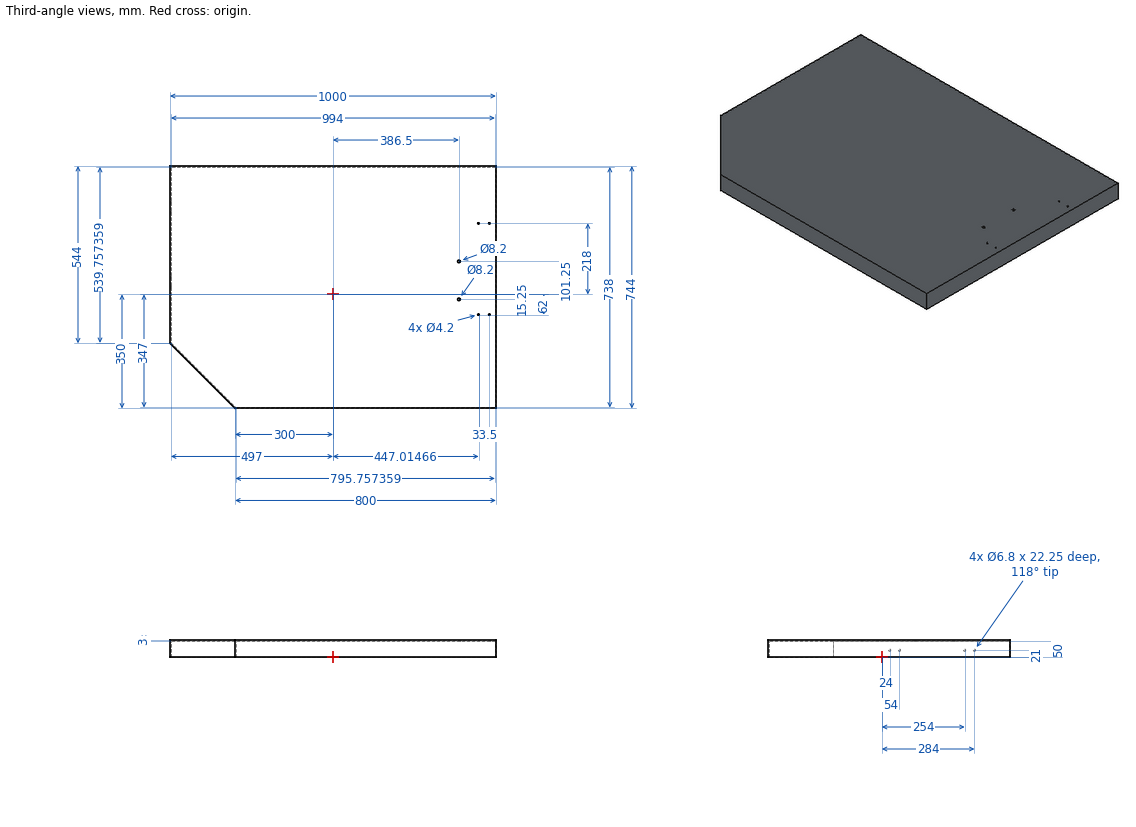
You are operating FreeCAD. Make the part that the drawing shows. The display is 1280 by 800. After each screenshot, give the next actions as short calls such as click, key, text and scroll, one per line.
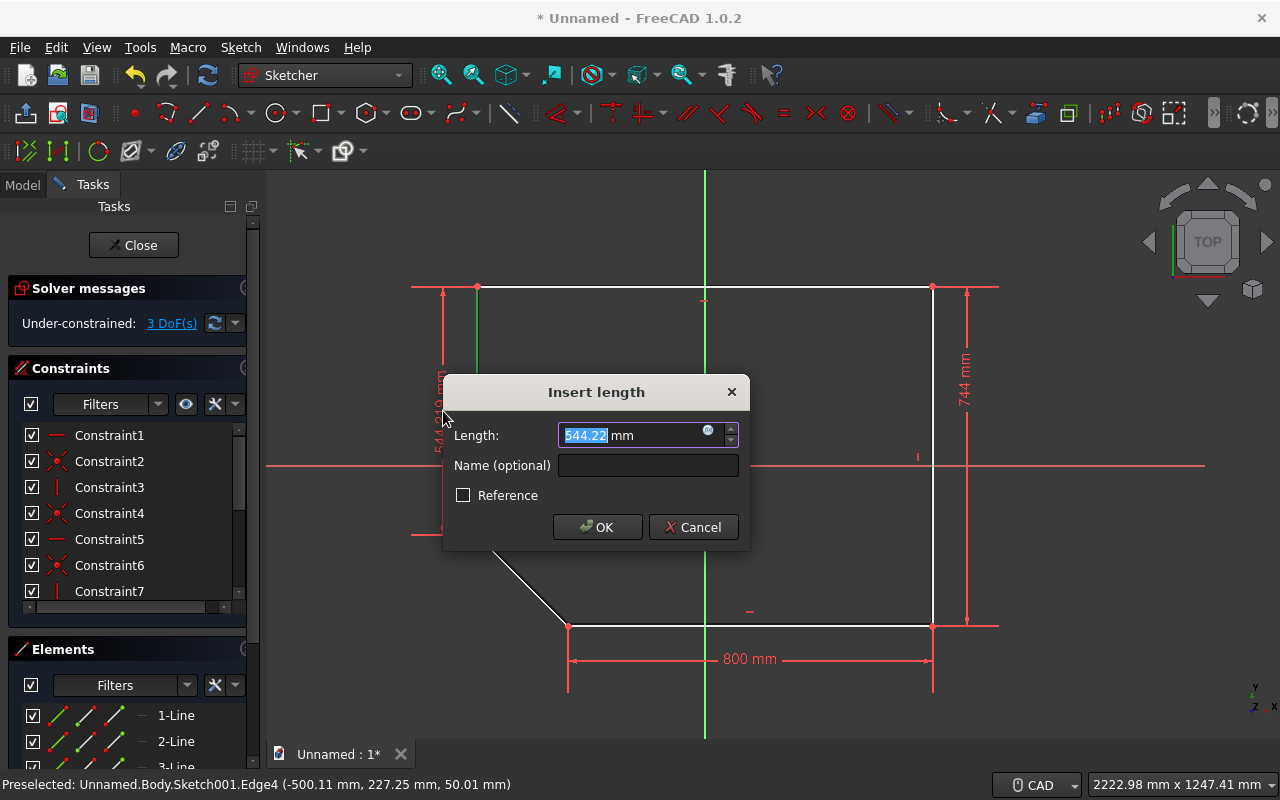
text(544)
key(Return)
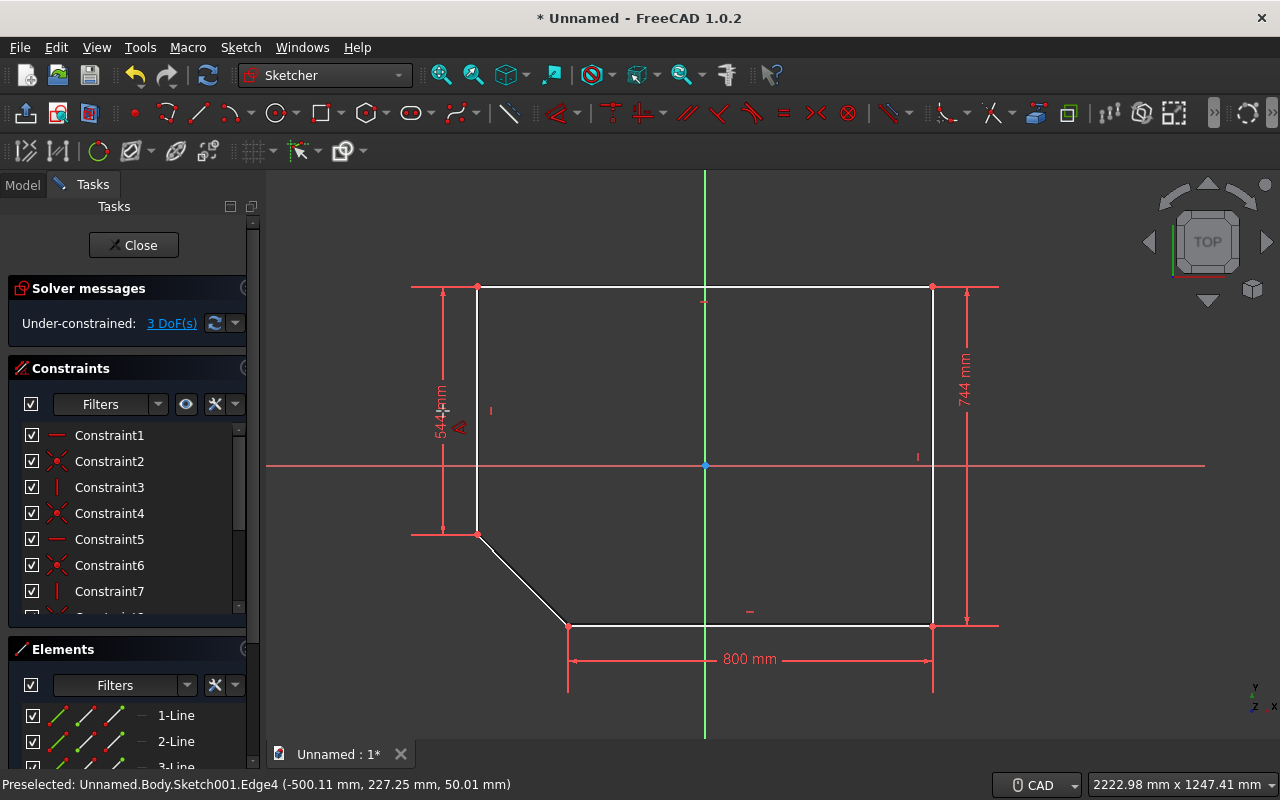
click(796, 287)
click(600, 253)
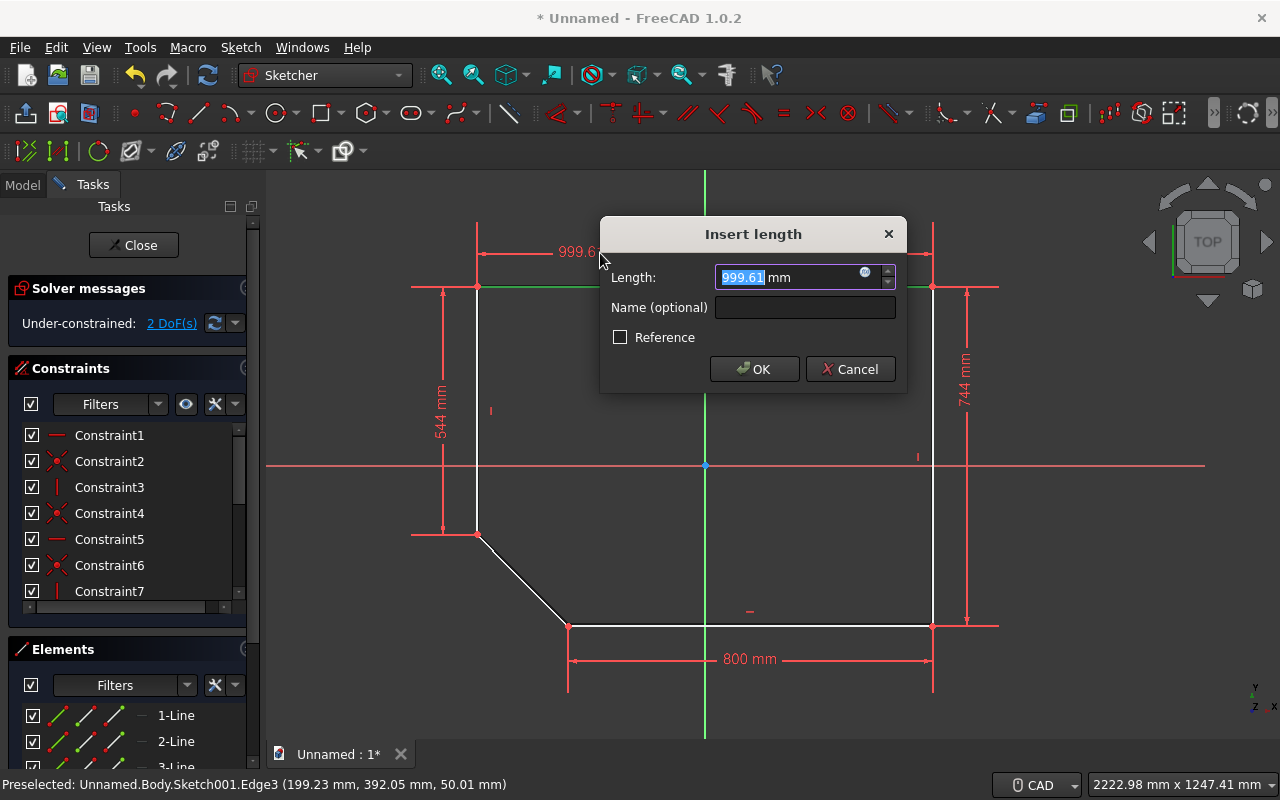
text(1000)
key(Return)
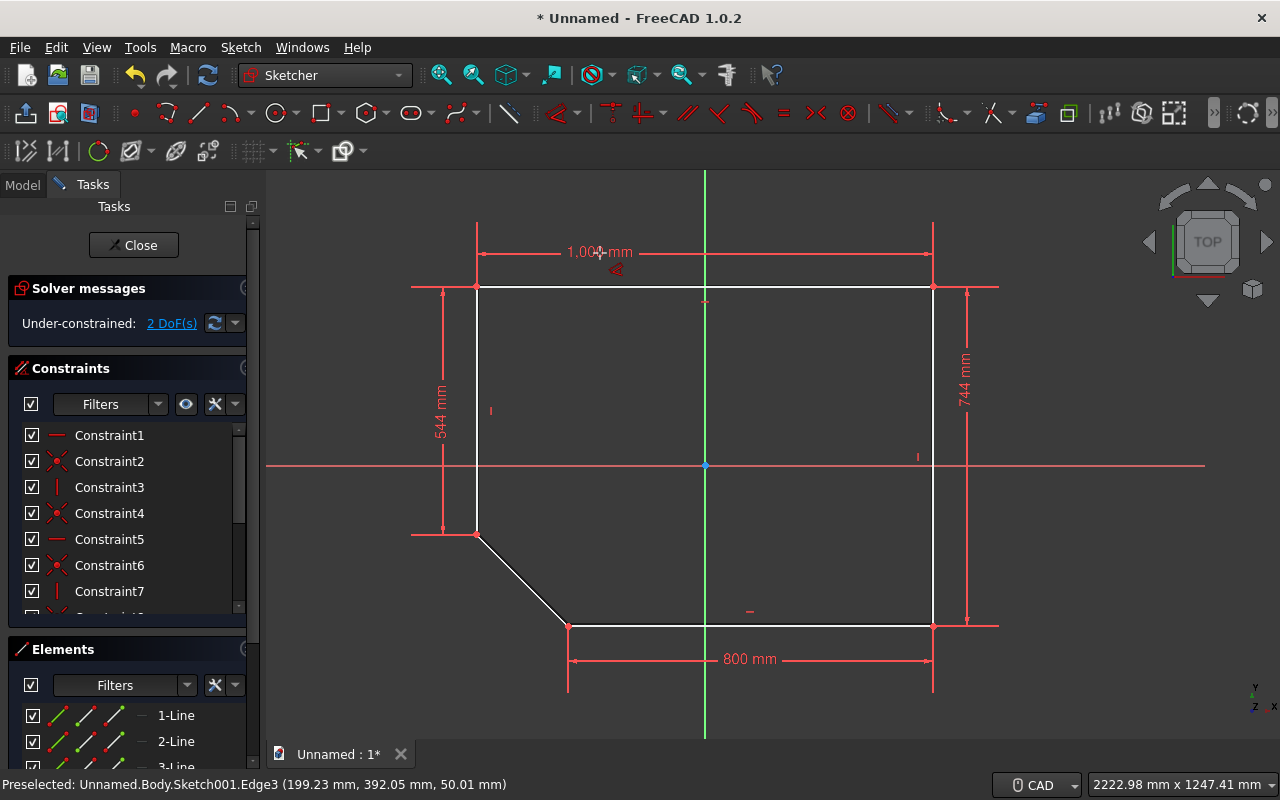
click(568, 626)
click(637, 660)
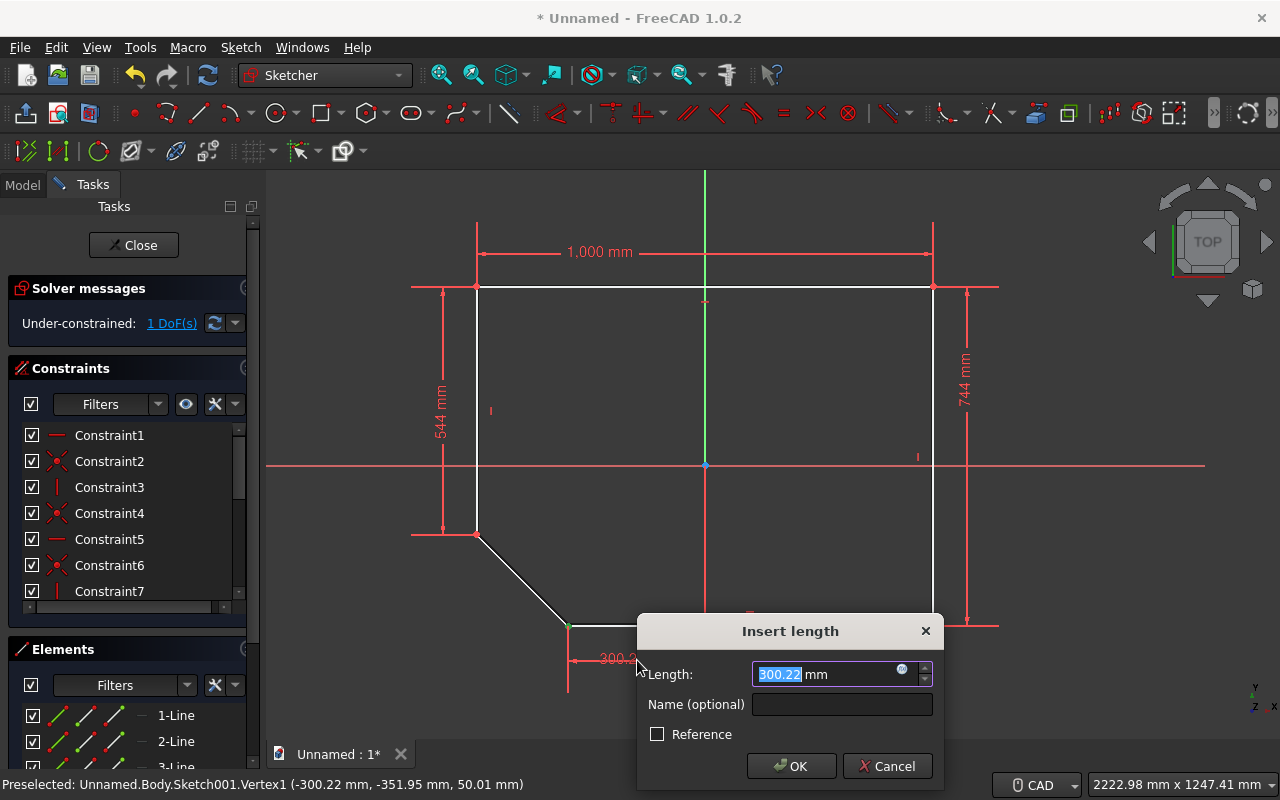
text(300)
key(Return)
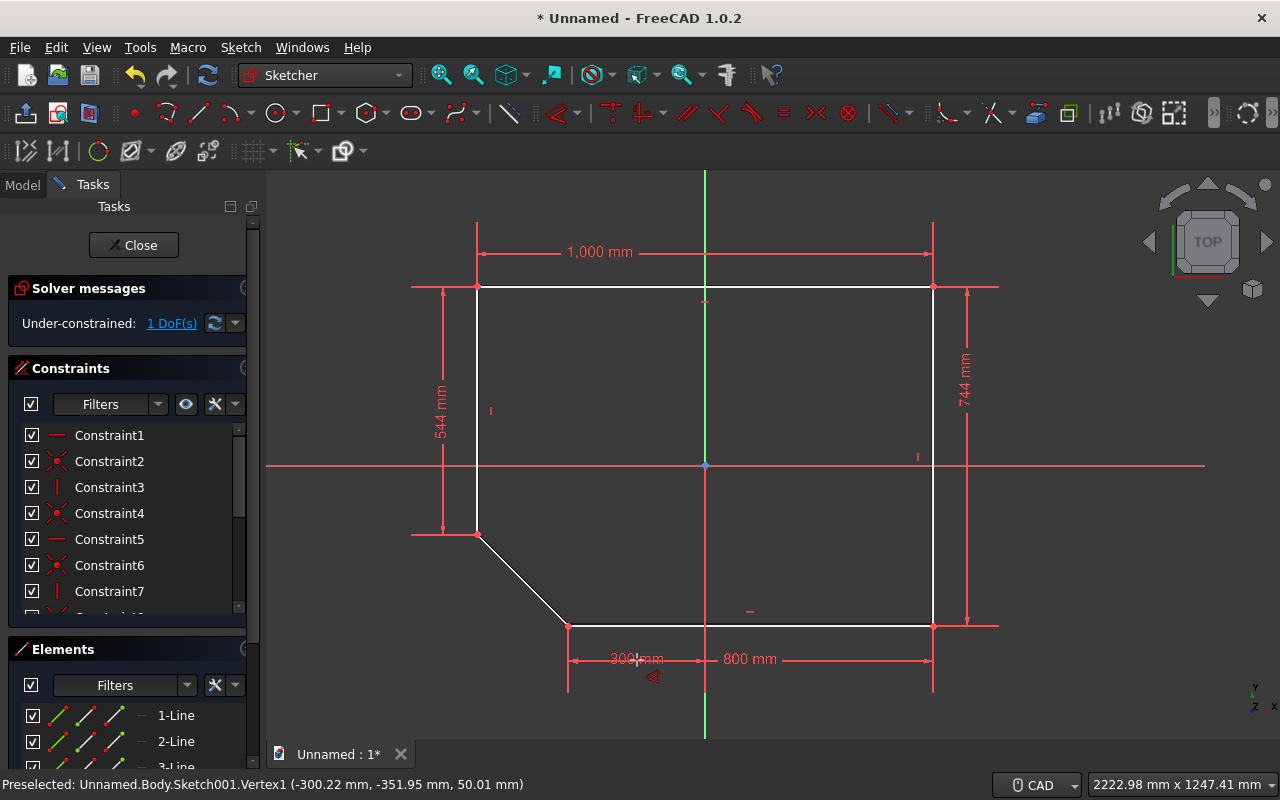
click(568, 626)
click(534, 546)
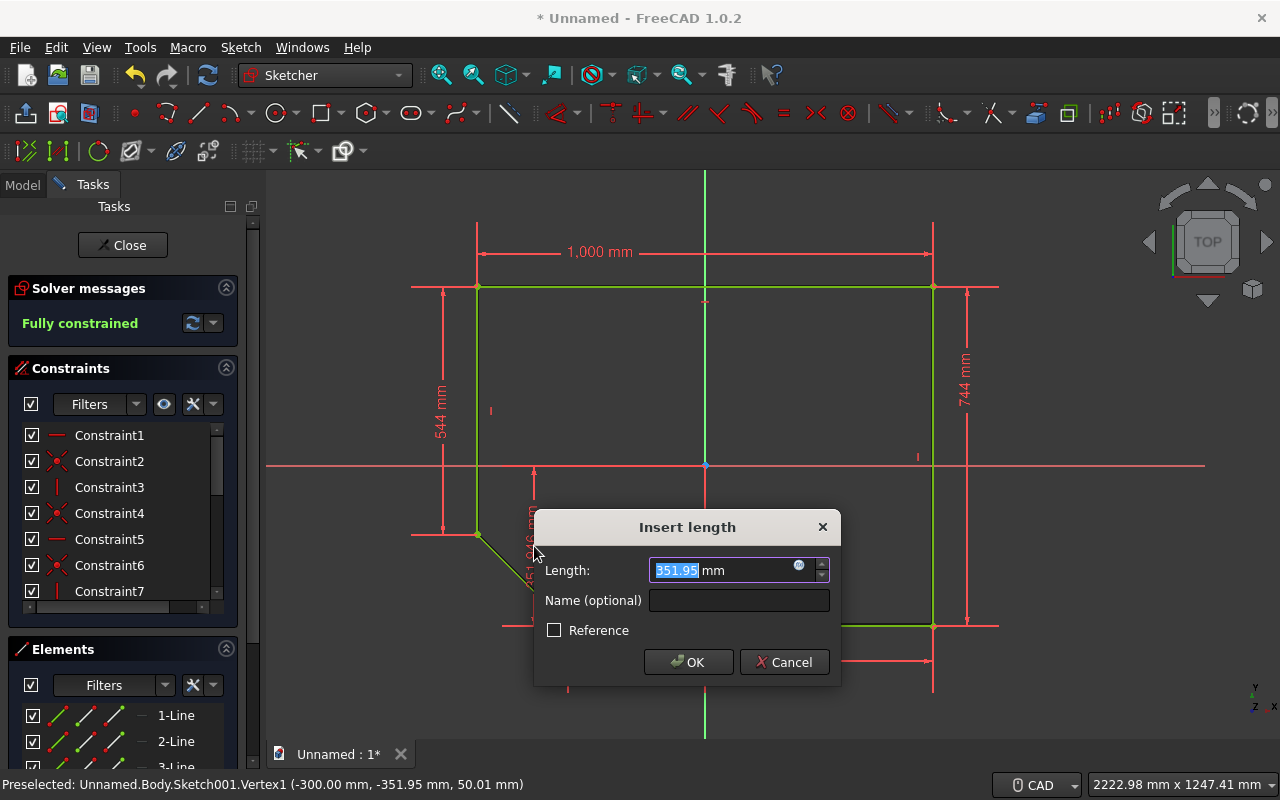
text(350)
key(Return)
key(Escape)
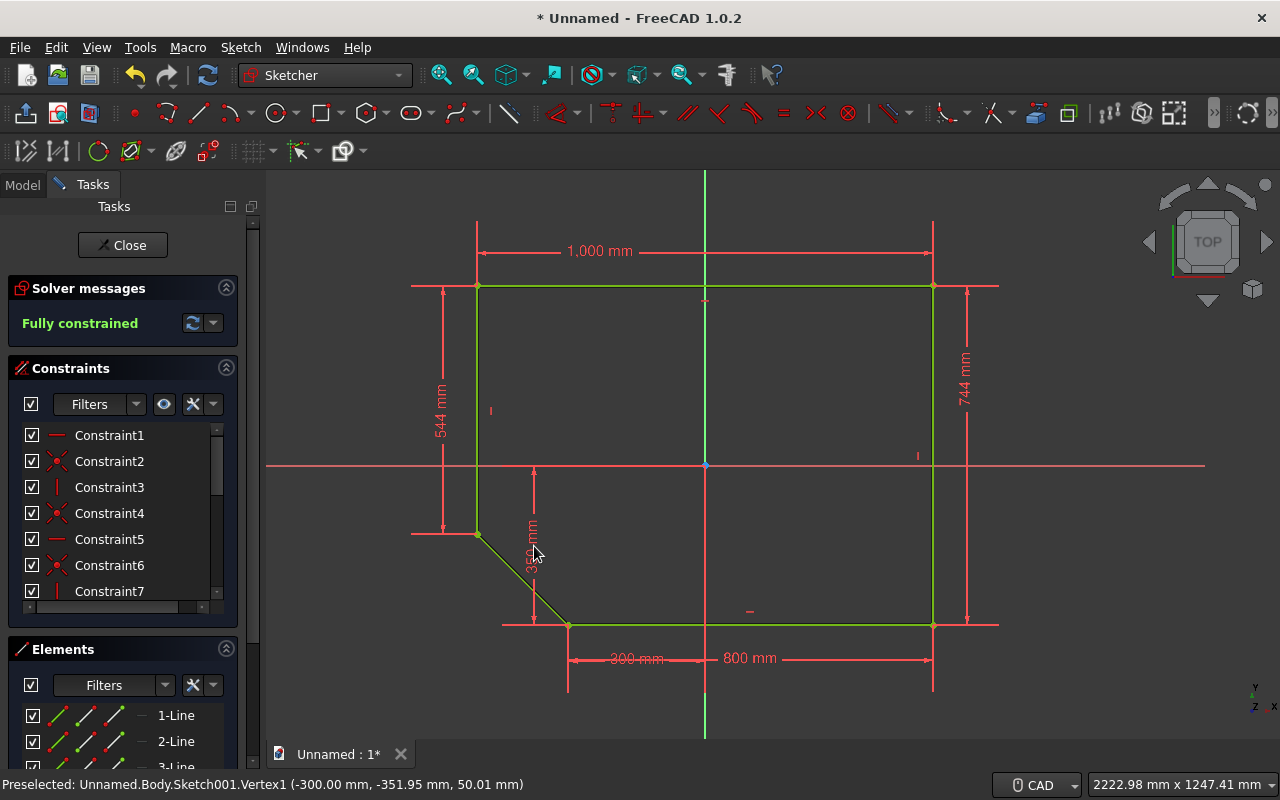
click(123, 245)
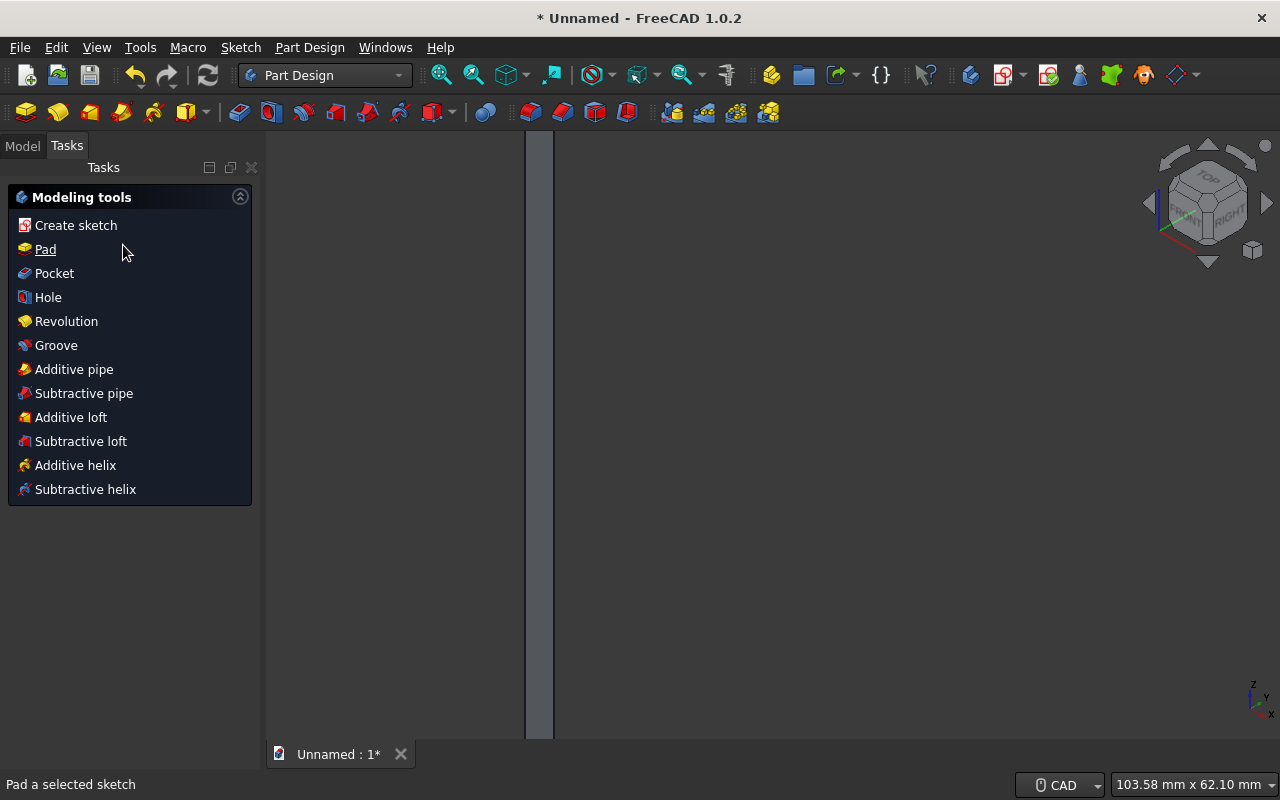
click(26, 112)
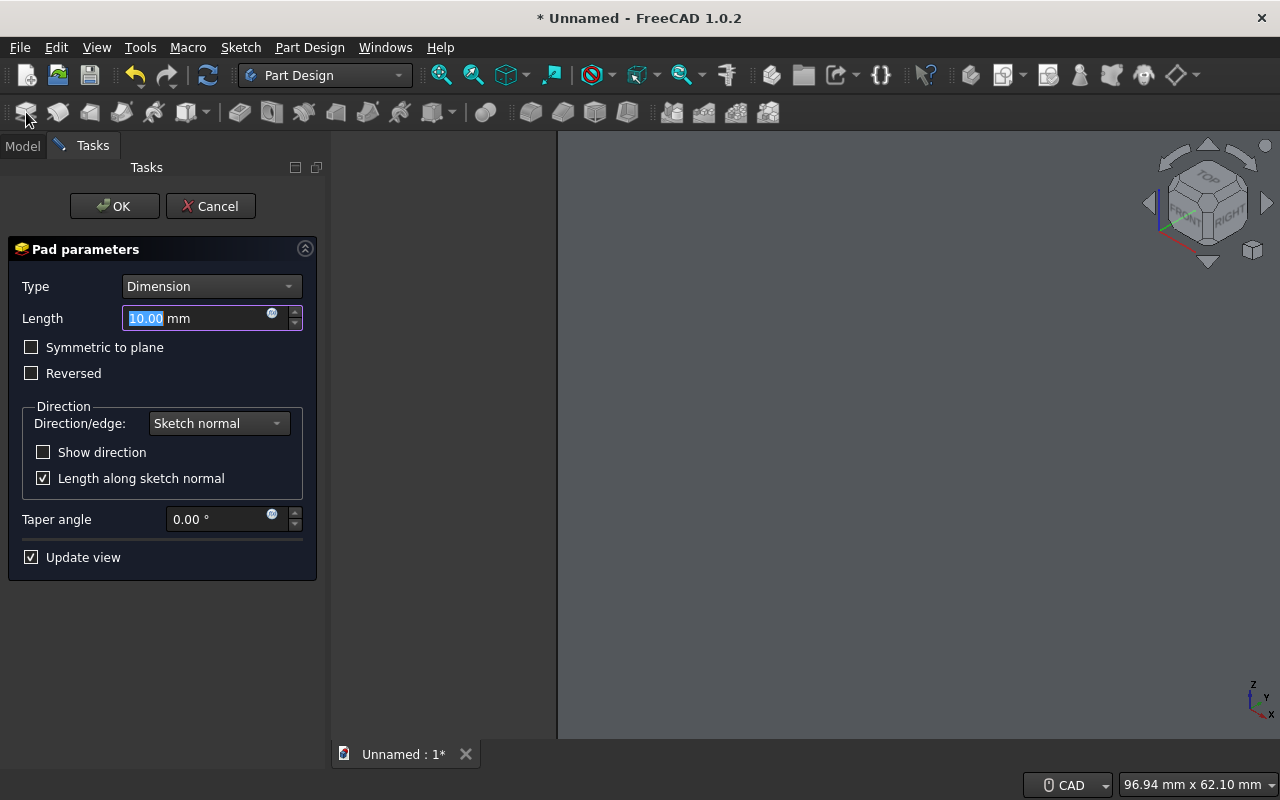
text(3)
key(Tab)